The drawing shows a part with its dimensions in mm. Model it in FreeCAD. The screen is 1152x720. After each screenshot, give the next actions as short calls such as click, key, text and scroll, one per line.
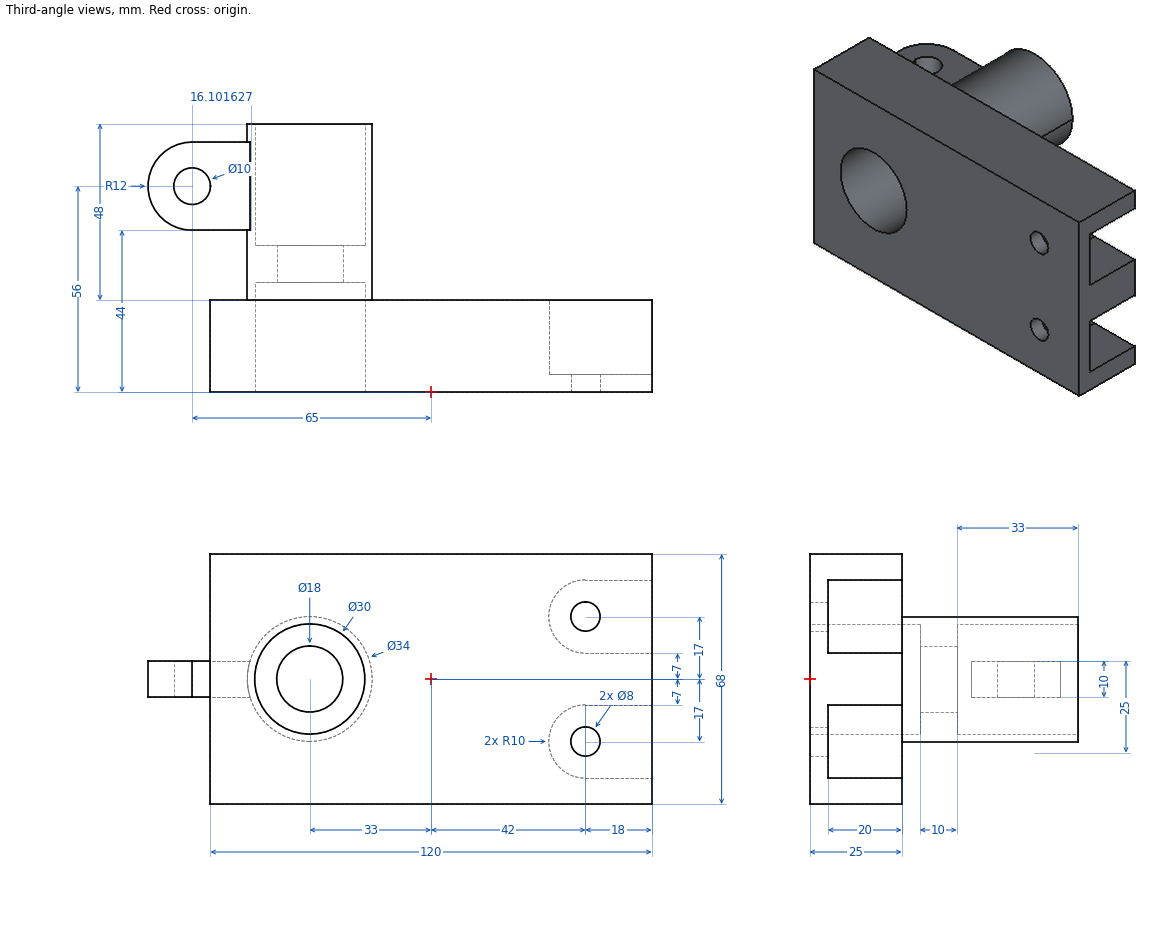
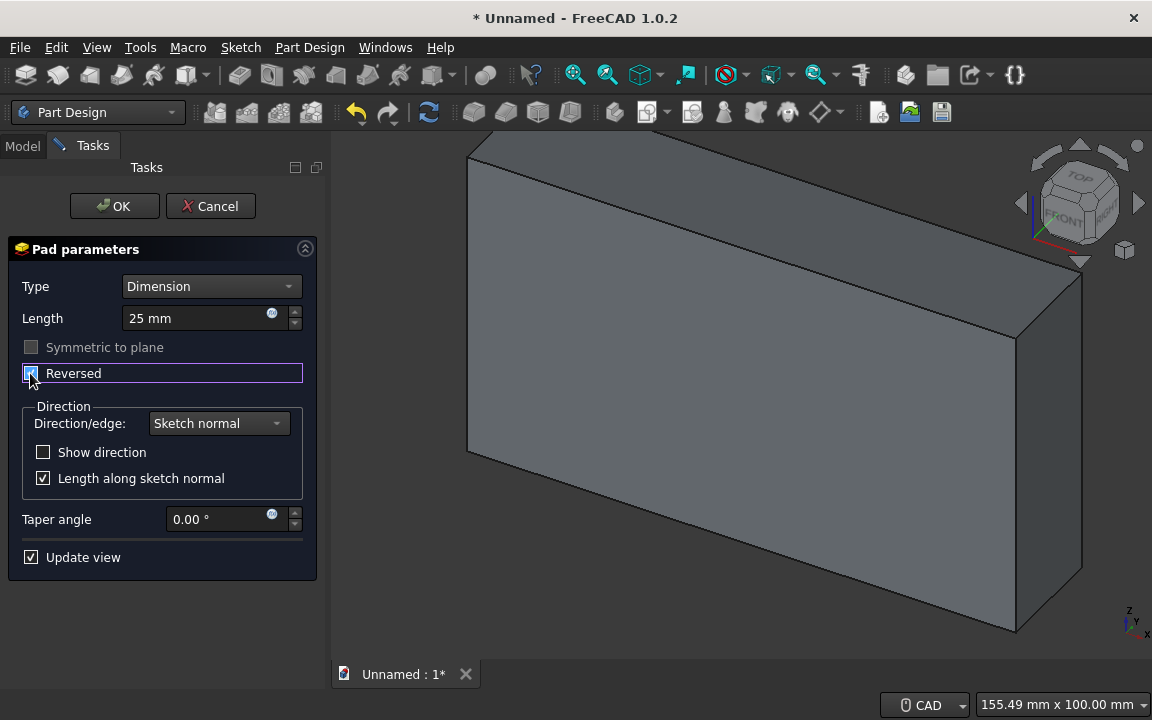
click(115, 206)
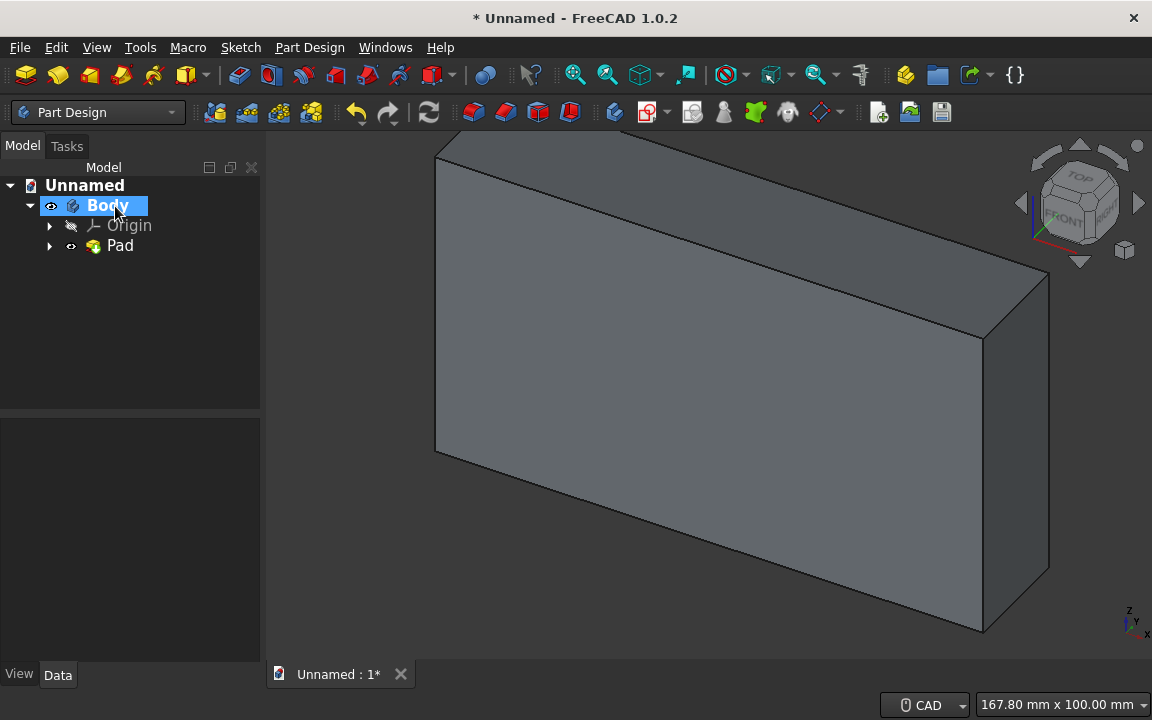
click(576, 76)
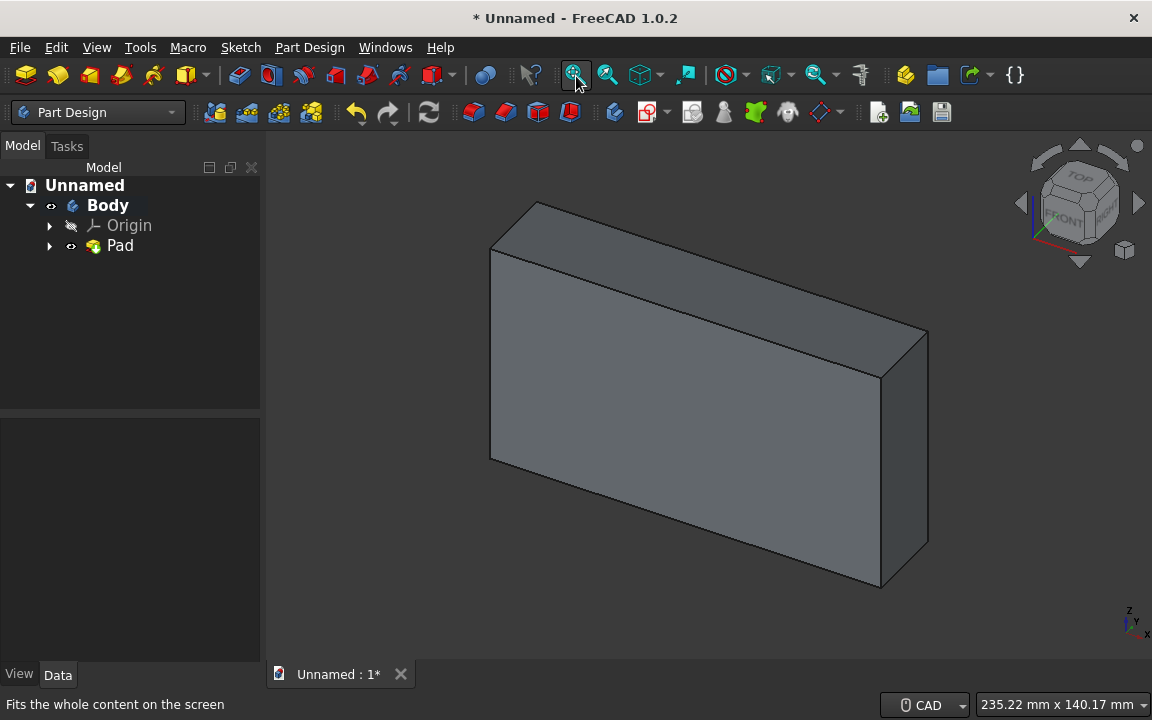
key(4)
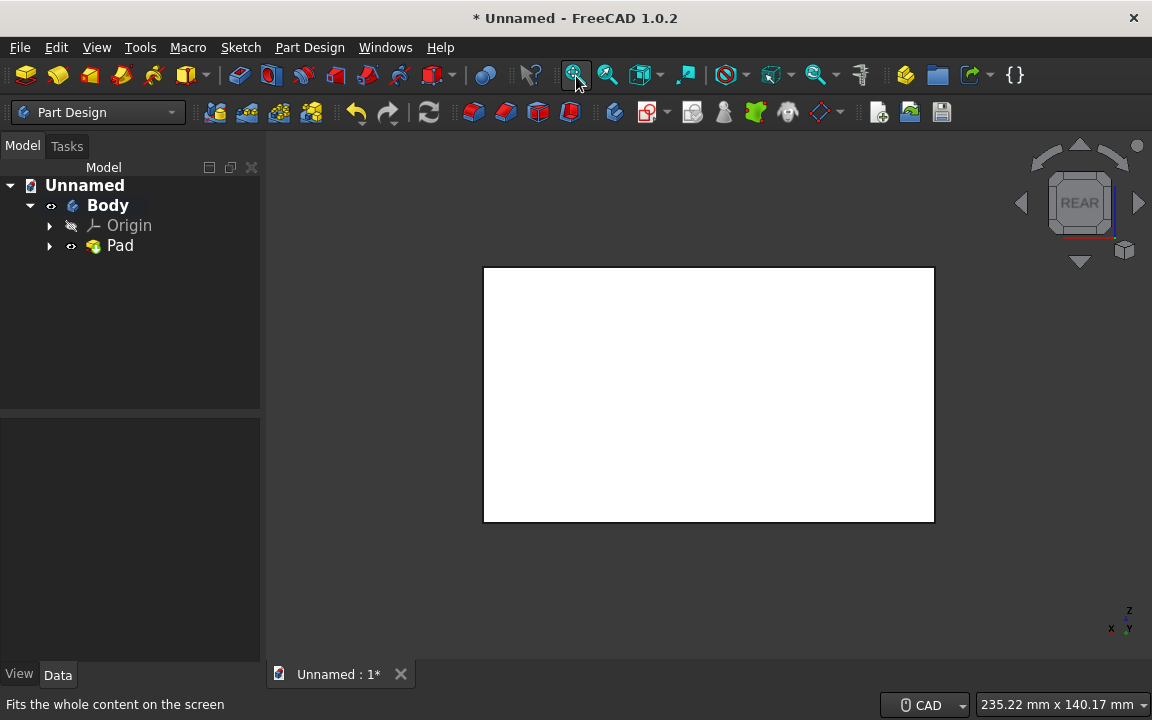
click(644, 394)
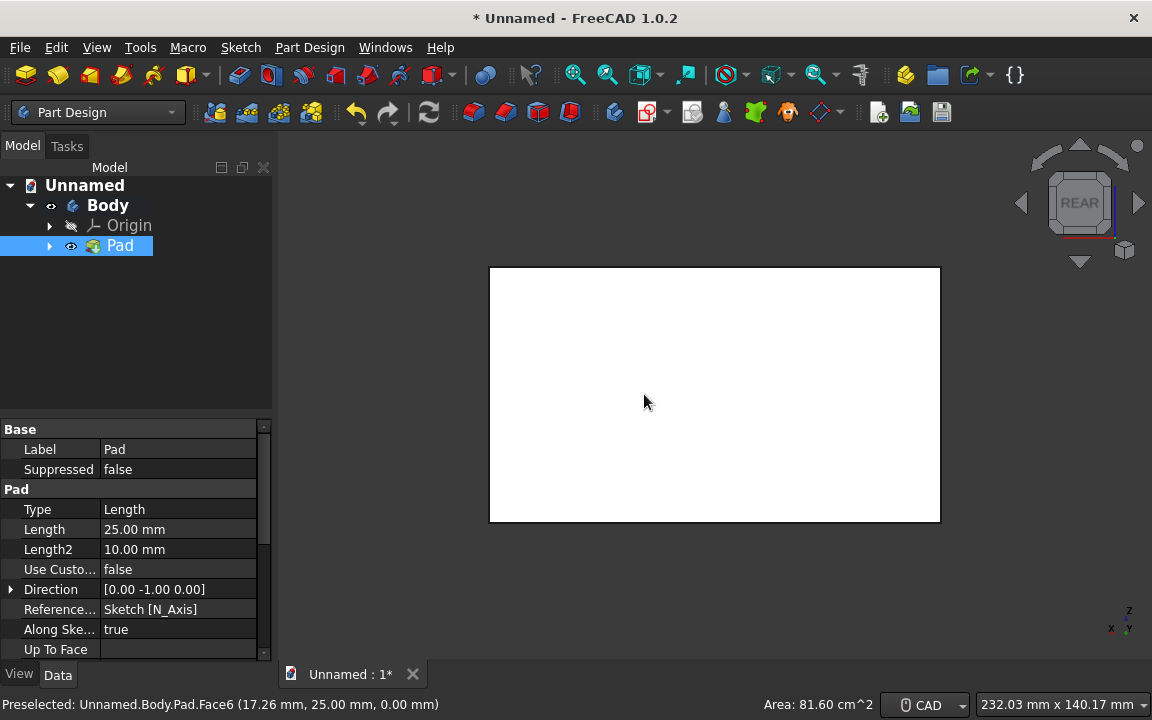
click(648, 112)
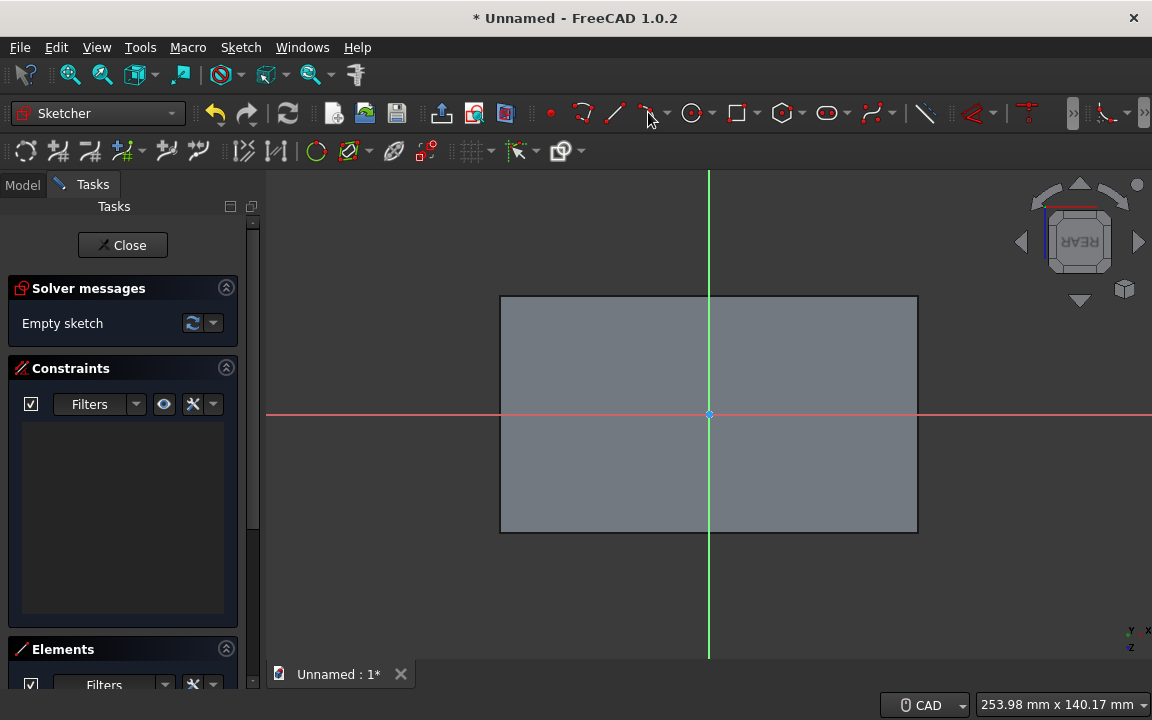
scroll(611, 415, up, 5)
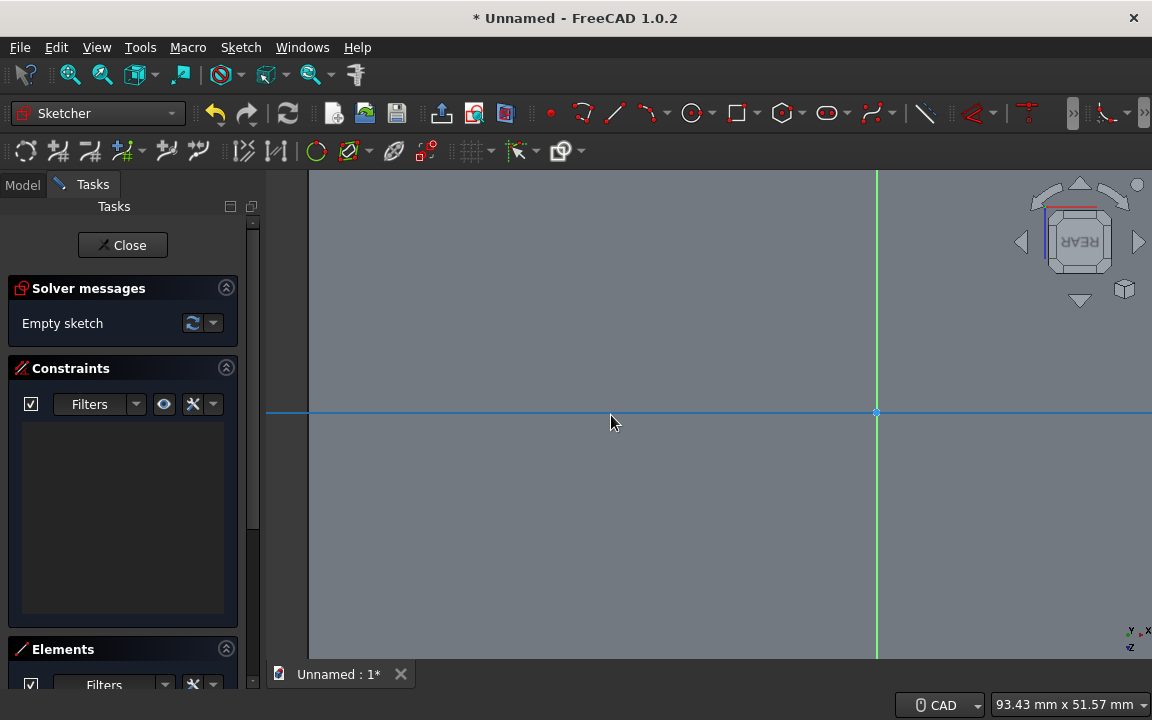
click(692, 114)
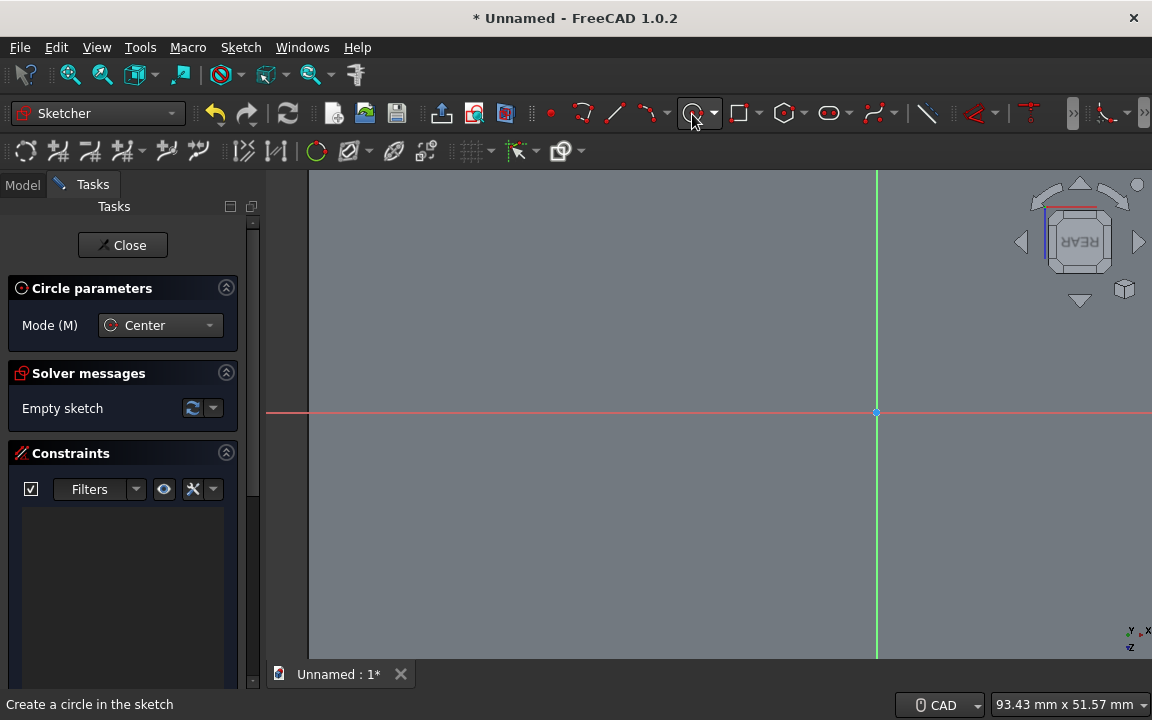
click(564, 413)
move(678, 299)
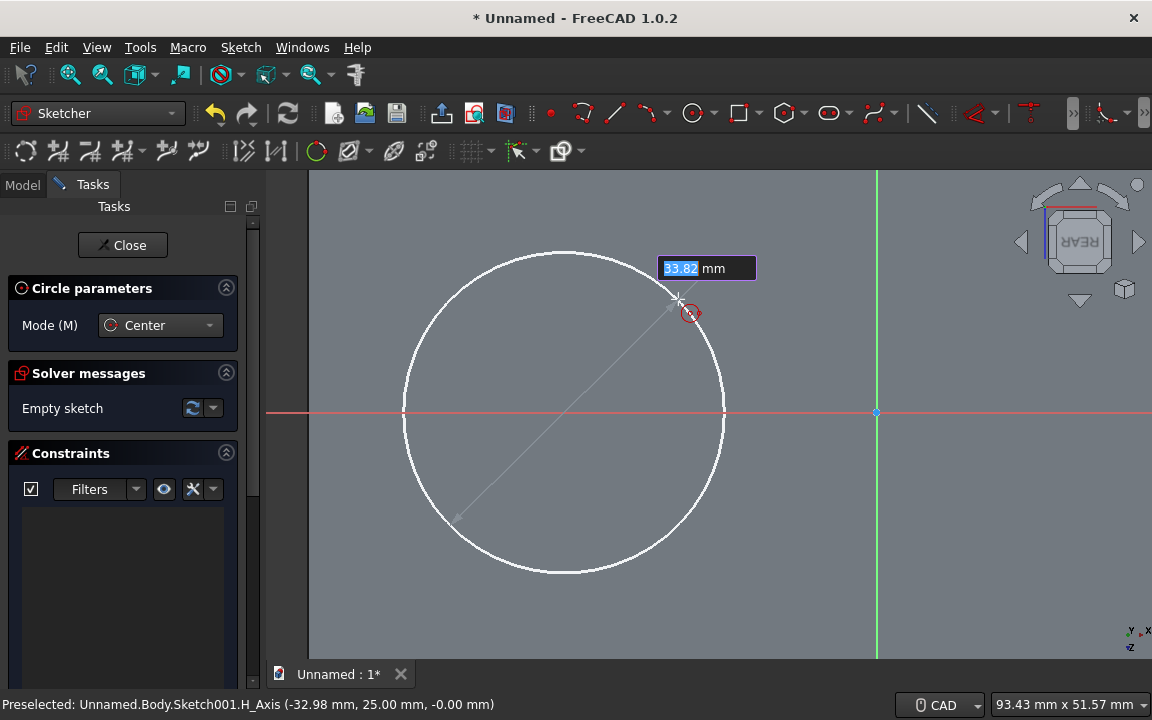
text(34)
key(Return)
key(Escape)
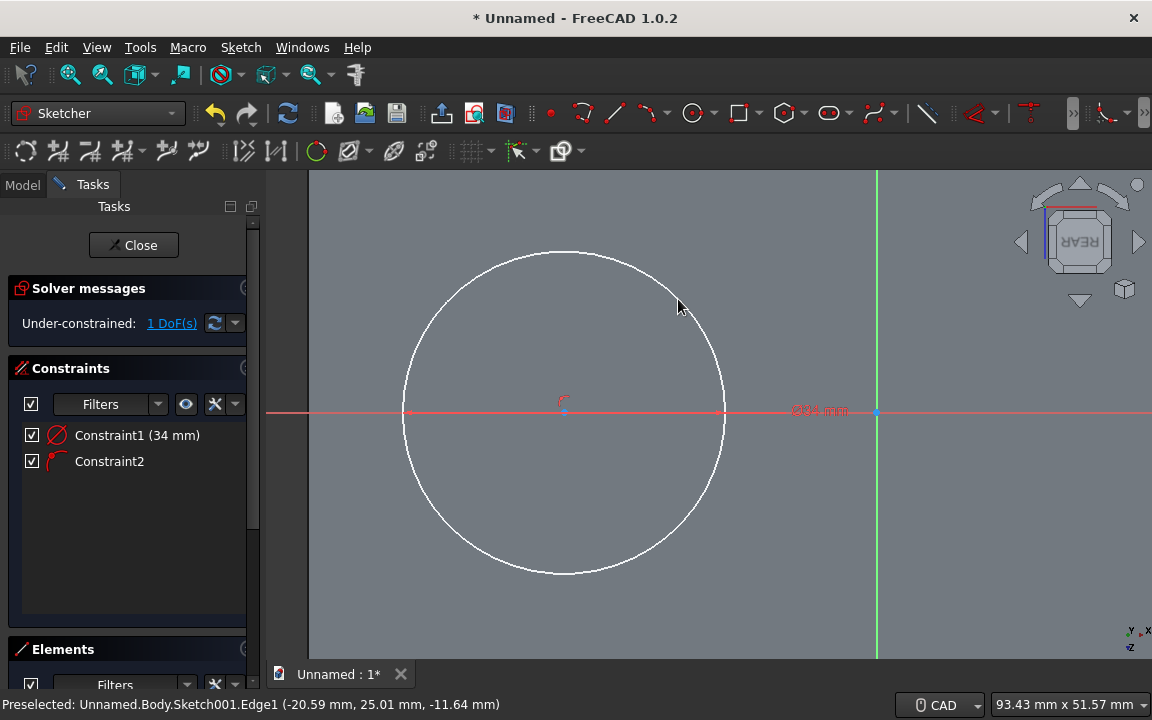
click(974, 114)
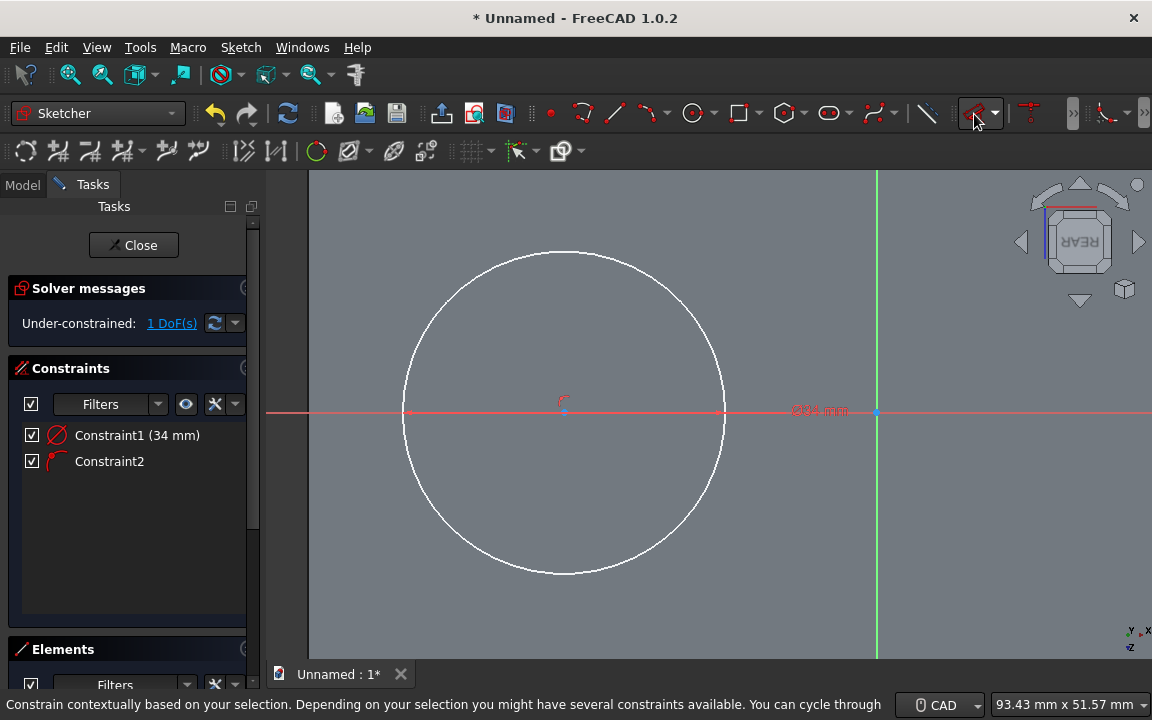
click(564, 413)
click(648, 447)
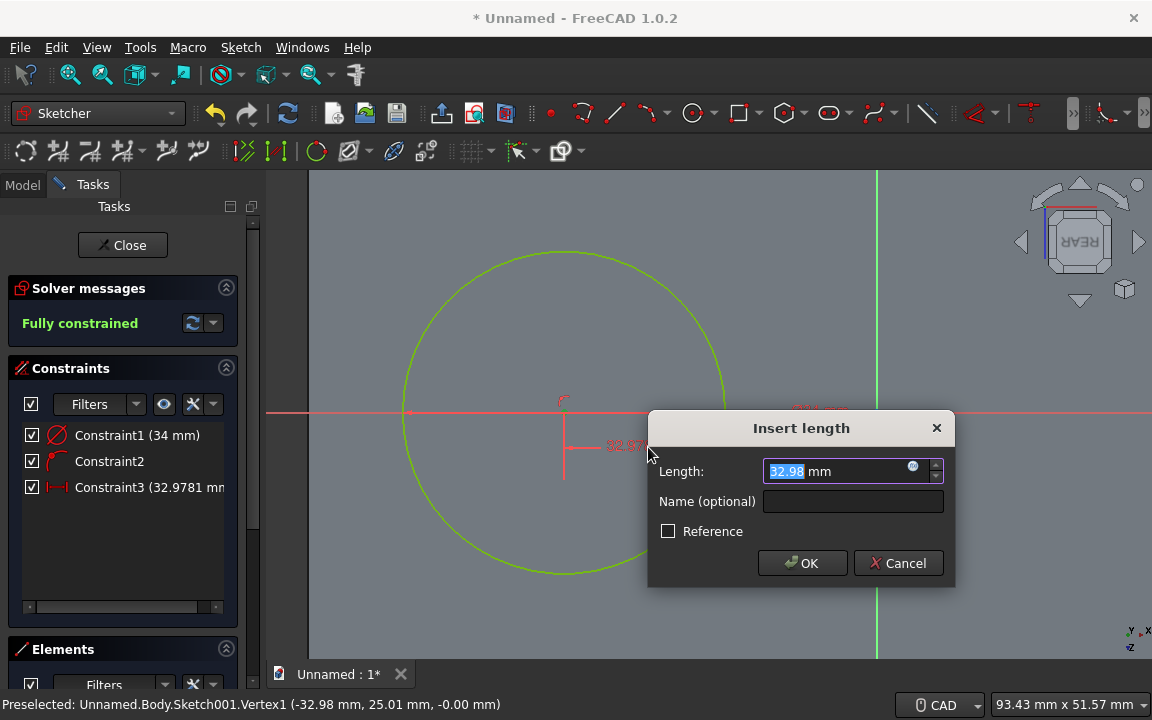
text(33)
key(Return)
key(Escape)